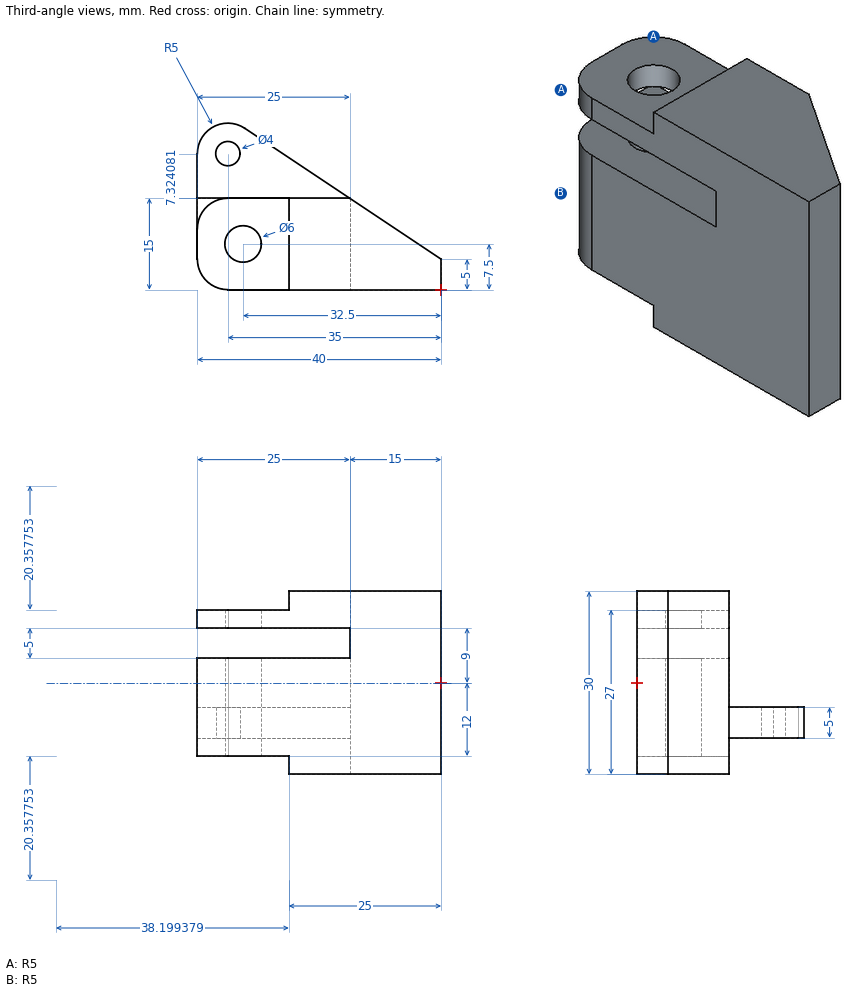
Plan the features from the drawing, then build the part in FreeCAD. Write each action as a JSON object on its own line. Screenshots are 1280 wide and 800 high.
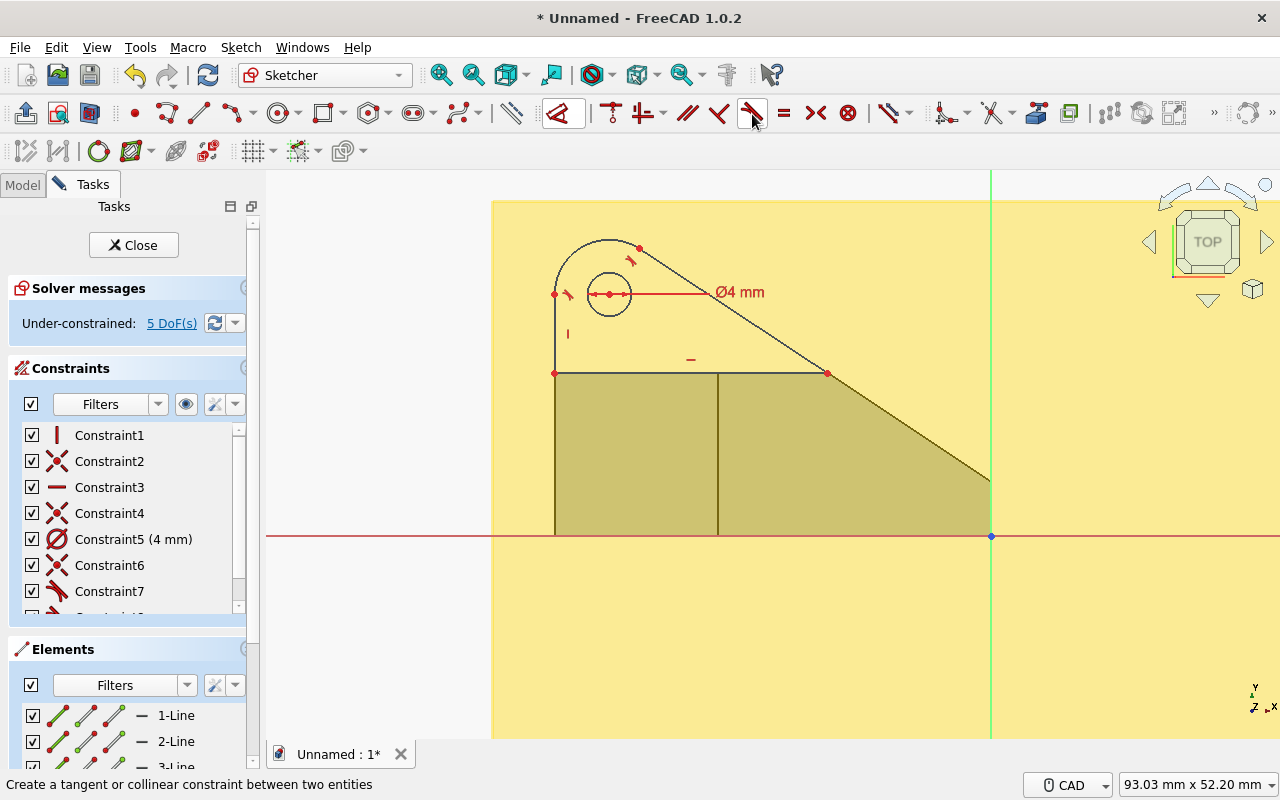
{"action": "left_click", "coordinate": [606, 240]}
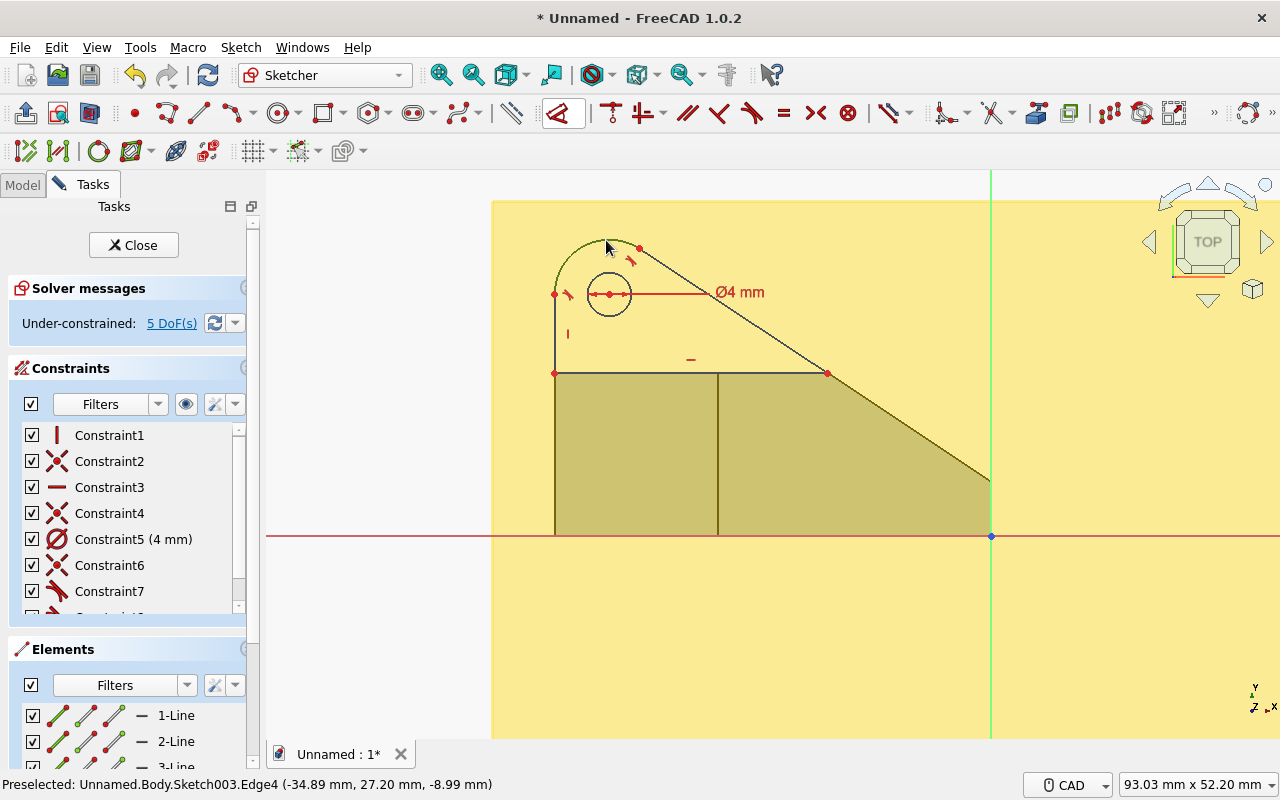
{"action": "left_click", "coordinate": [580, 114]}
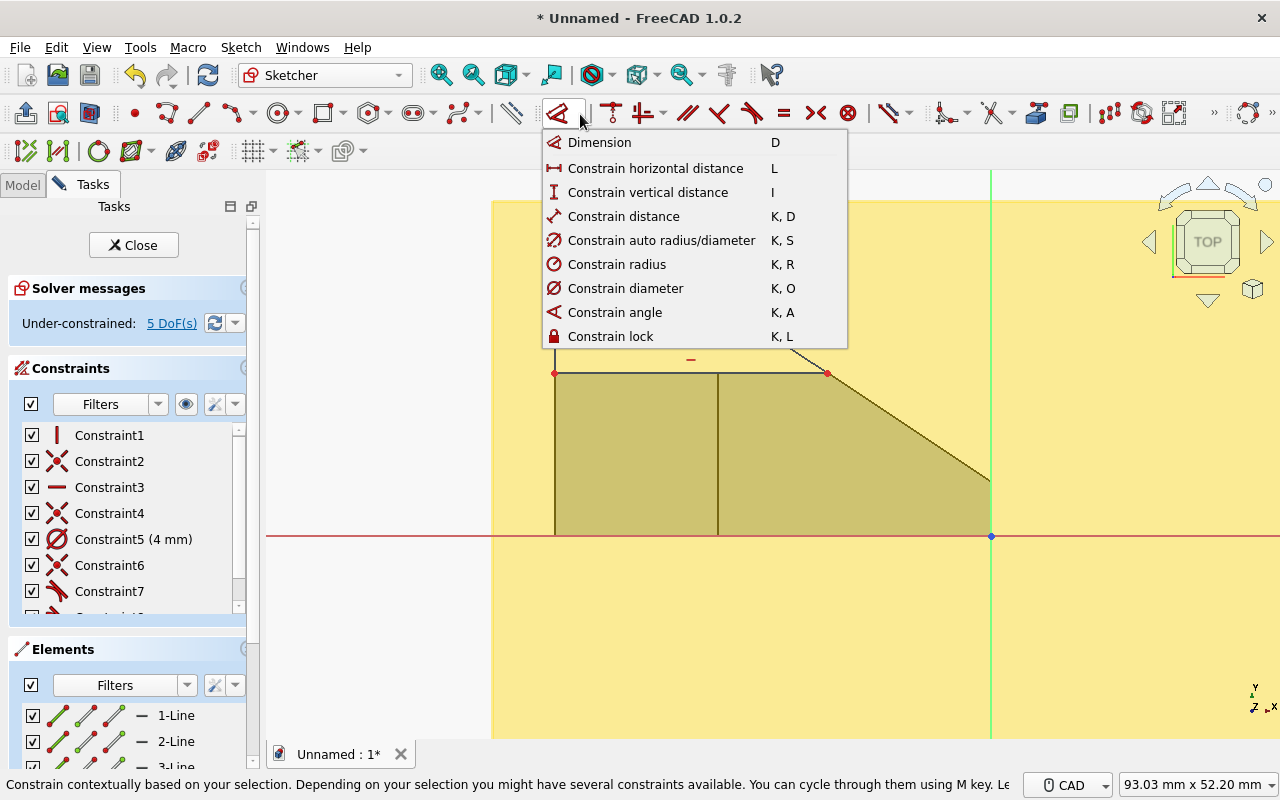
{"action": "left_click", "coordinate": [695, 264]}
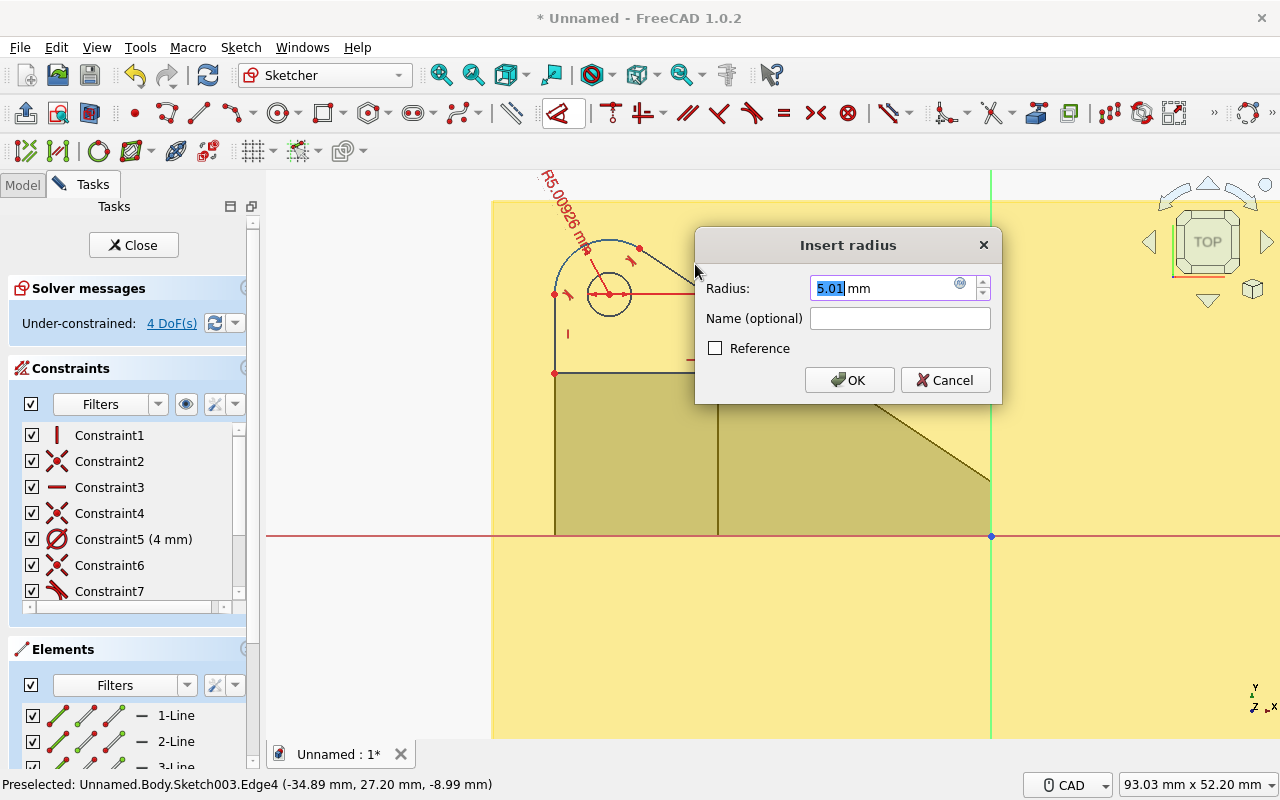
{"action": "type", "text": "5"}
{"action": "key", "text": "Return"}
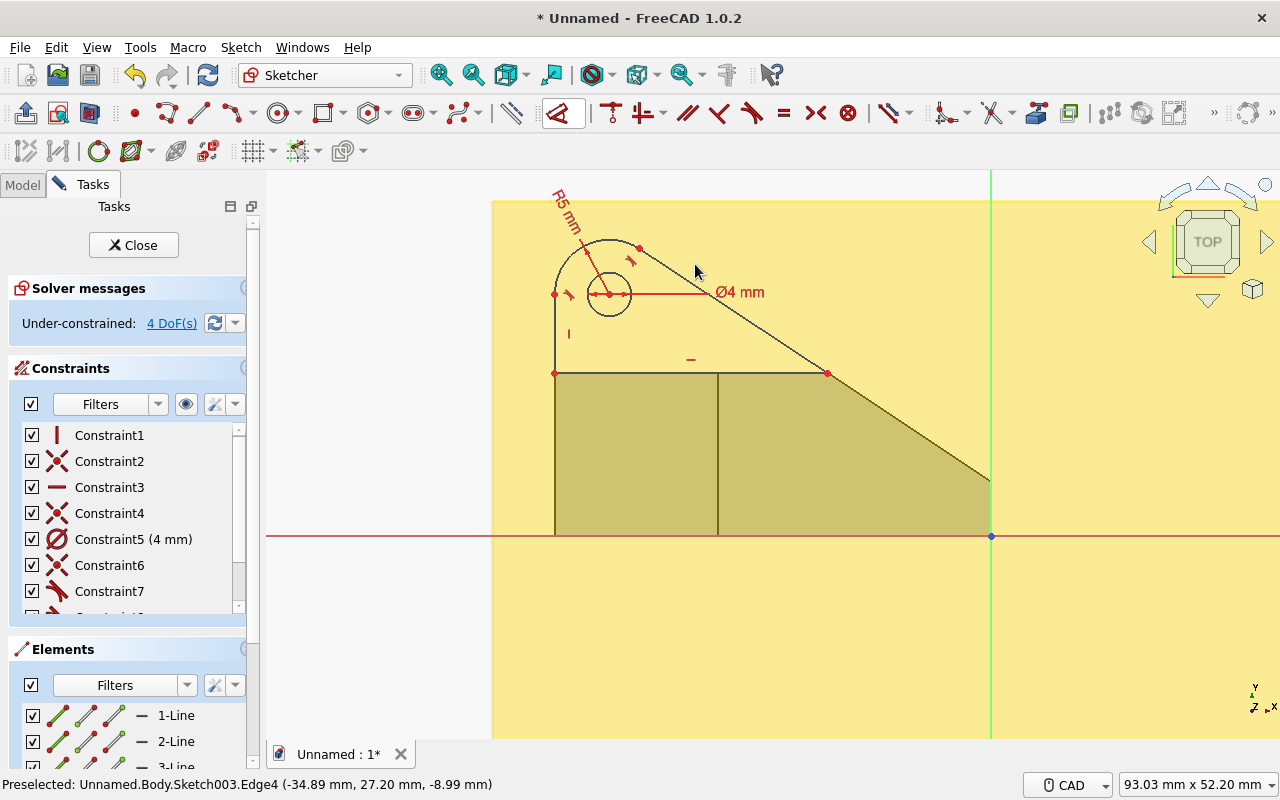
{"action": "left_click", "coordinate": [637, 373]}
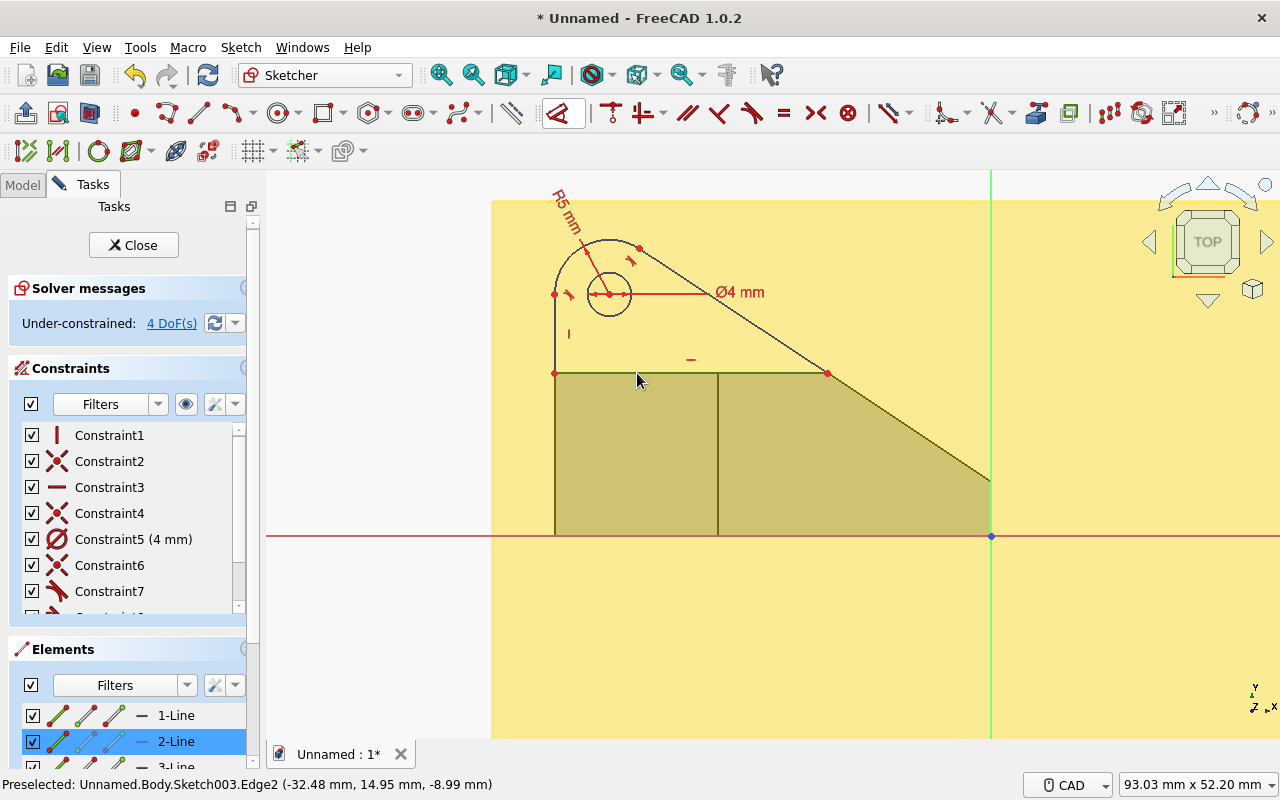
{"action": "key", "text": "l"}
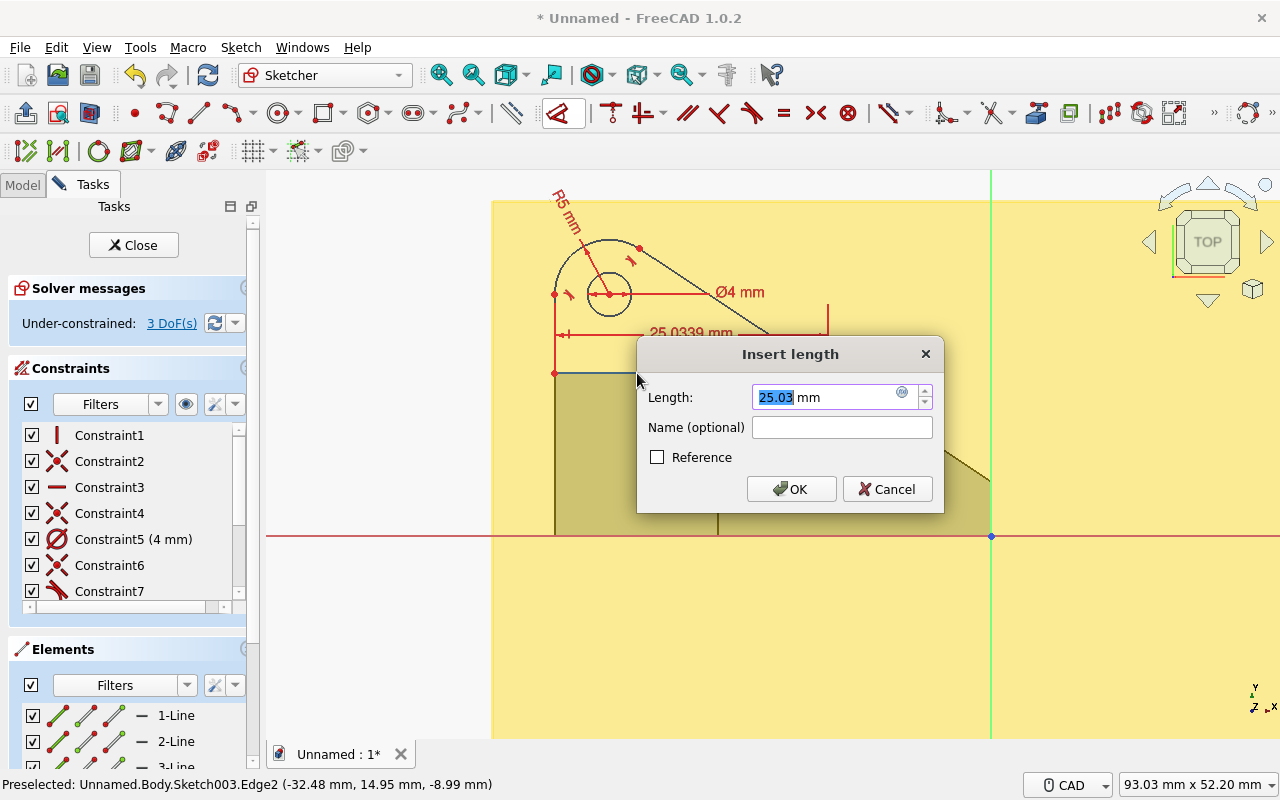
{"action": "type", "text": "25"}
{"action": "key", "text": "Return"}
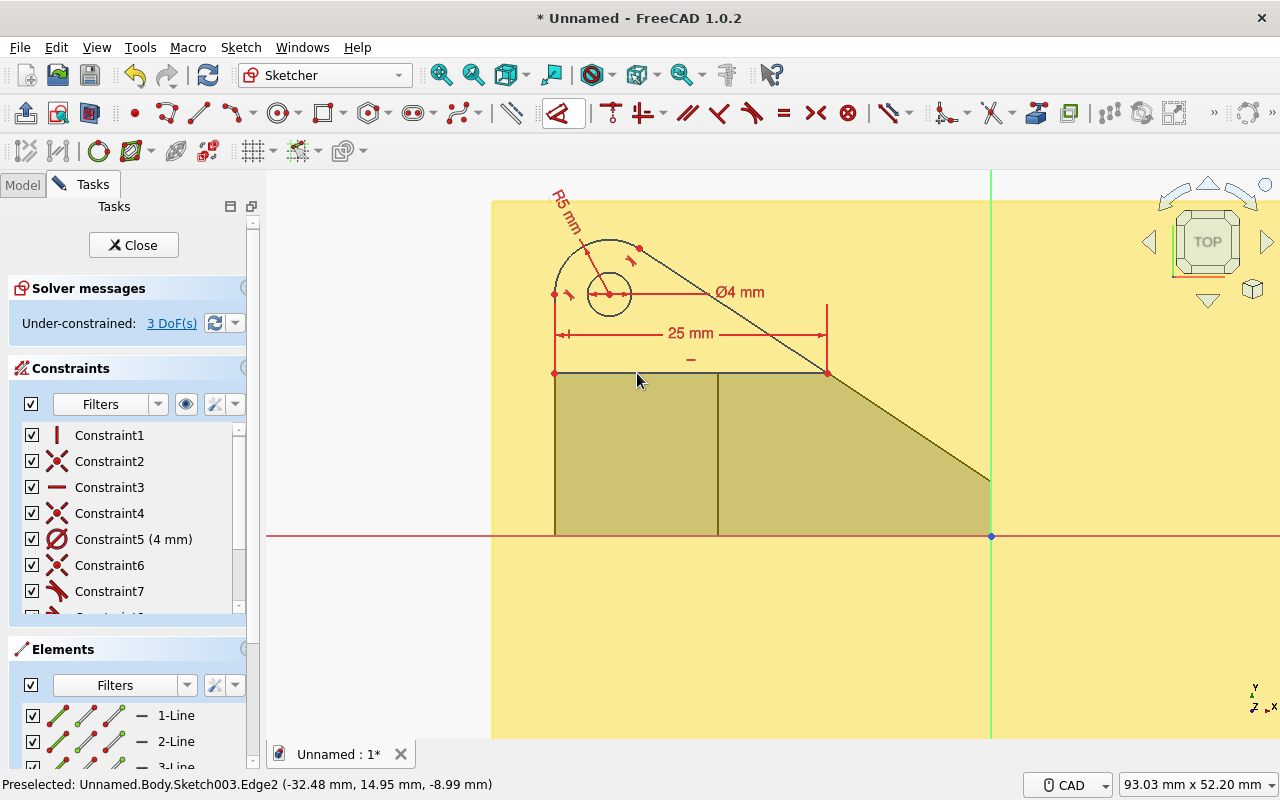
{"action": "left_click", "coordinate": [609, 294]}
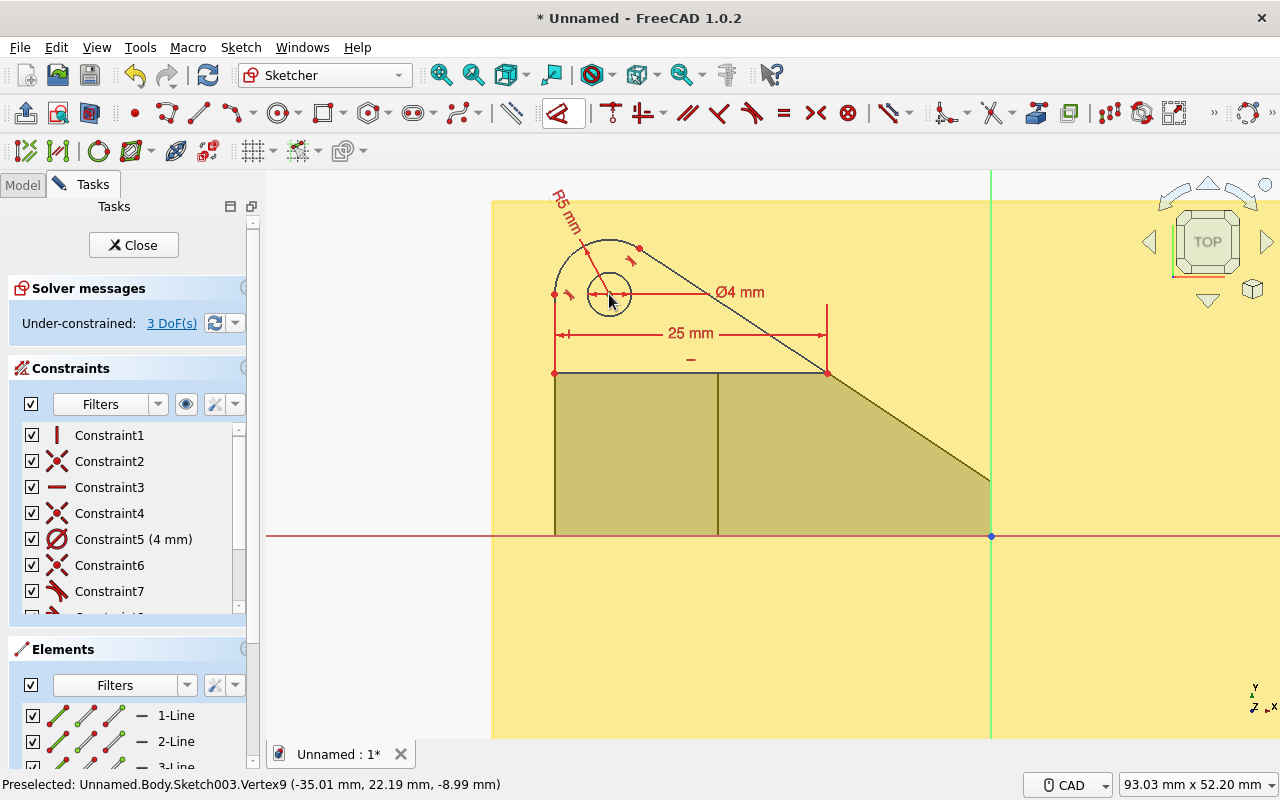
{"action": "key", "text": "l"}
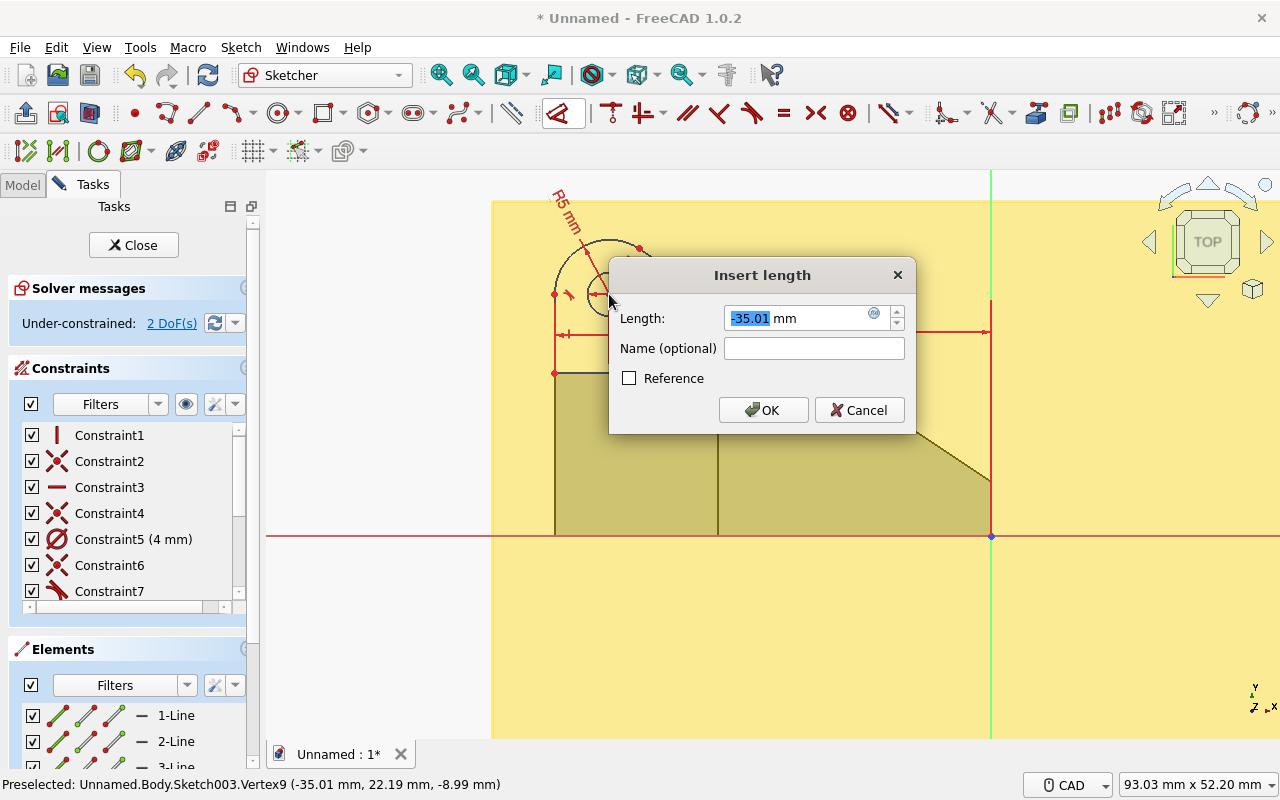
{"action": "type", "text": "-35"}
{"action": "key", "text": "Return"}